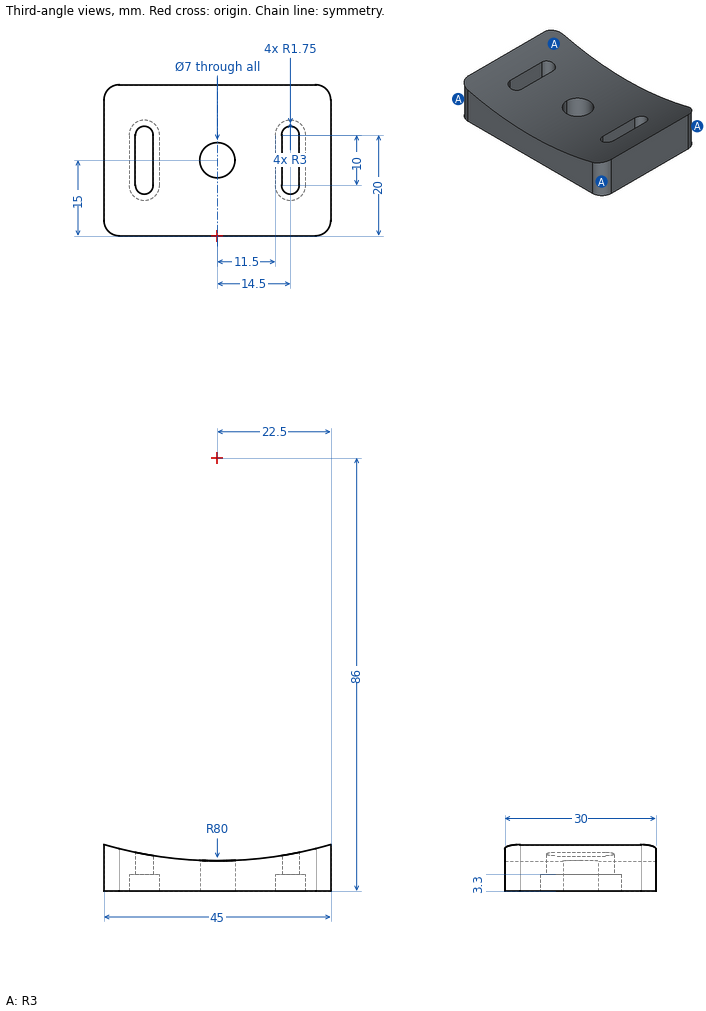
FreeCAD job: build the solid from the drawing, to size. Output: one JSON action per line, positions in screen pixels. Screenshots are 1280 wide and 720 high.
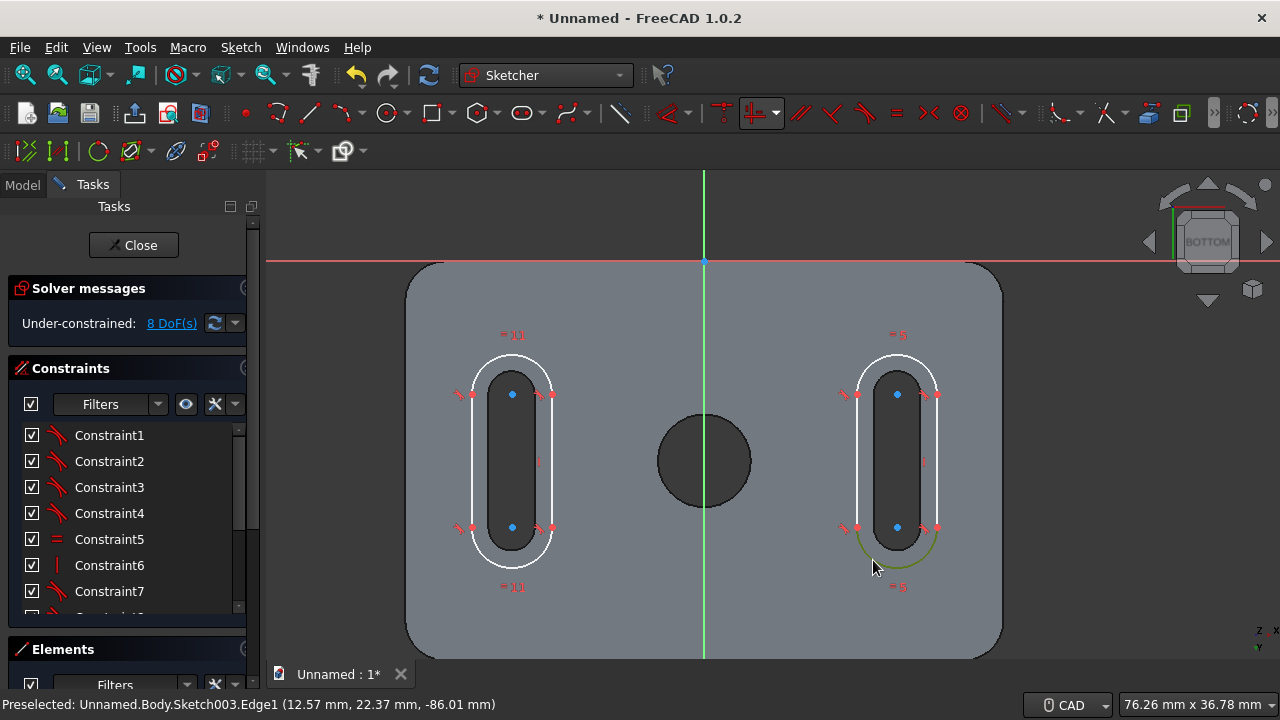
{"action": "left_click", "coordinate": [488, 560]}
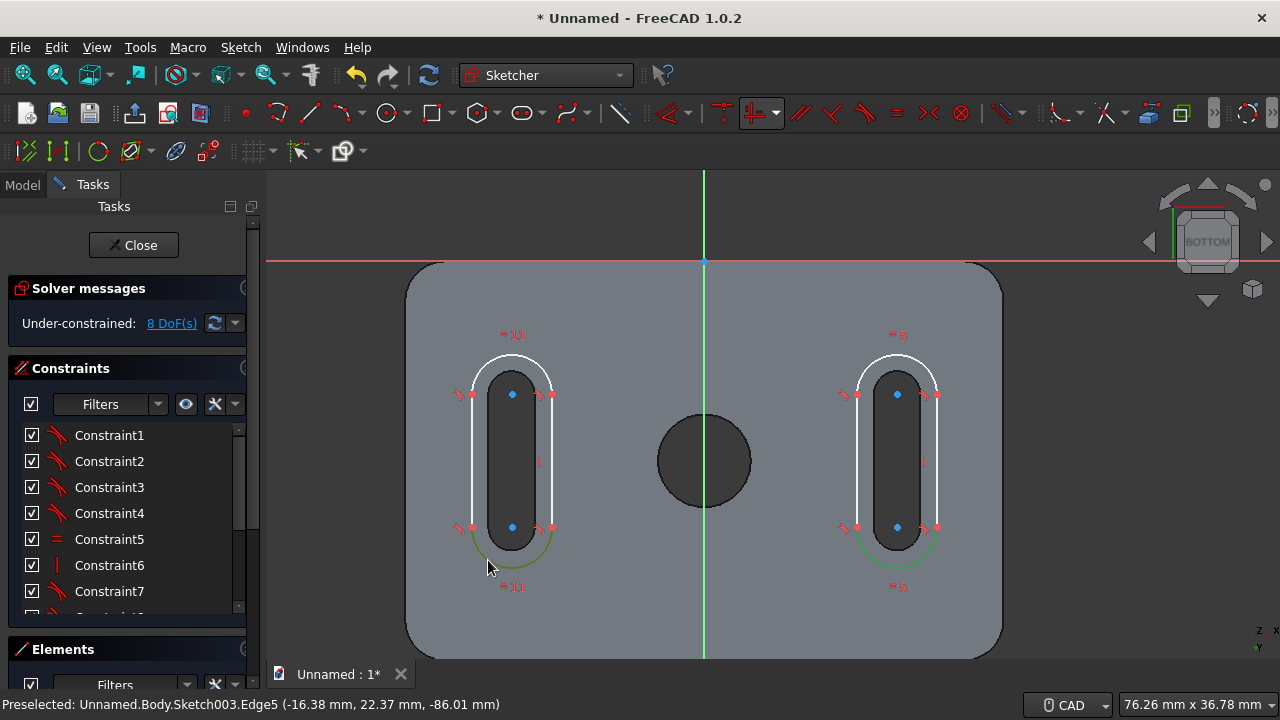
{"action": "left_click", "coordinate": [898, 114]}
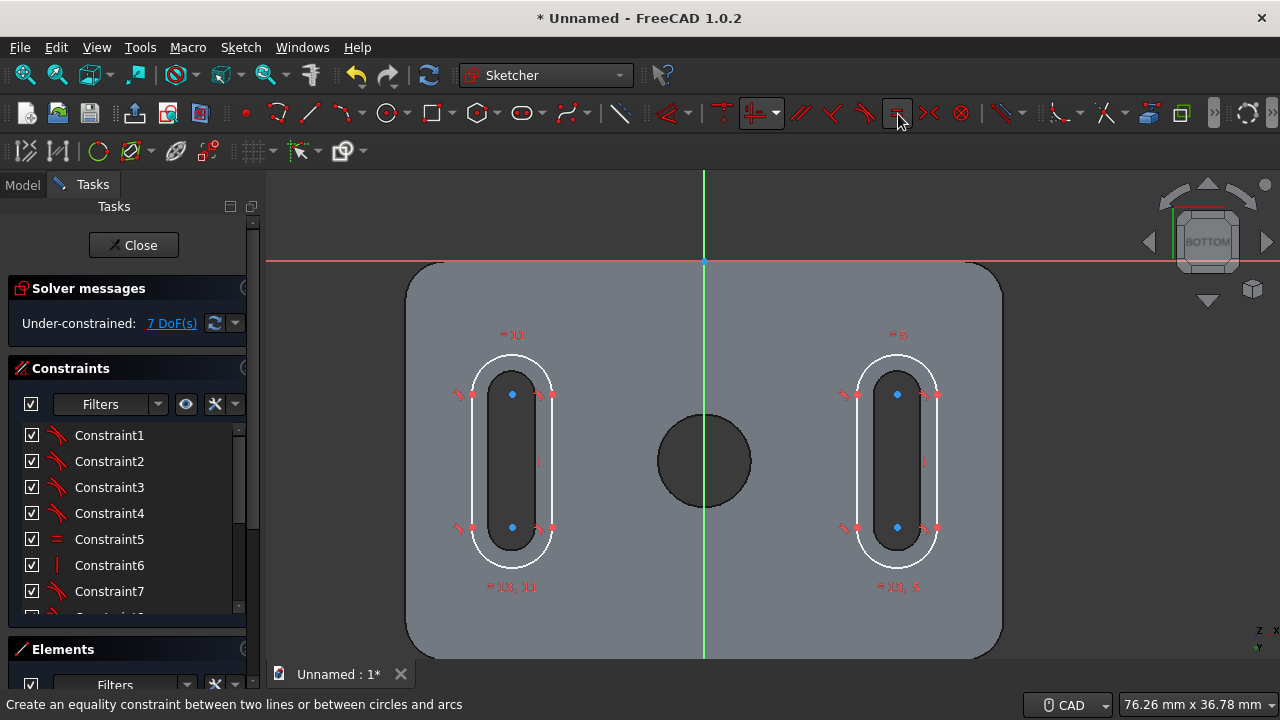
{"action": "left_click", "coordinate": [897, 528]}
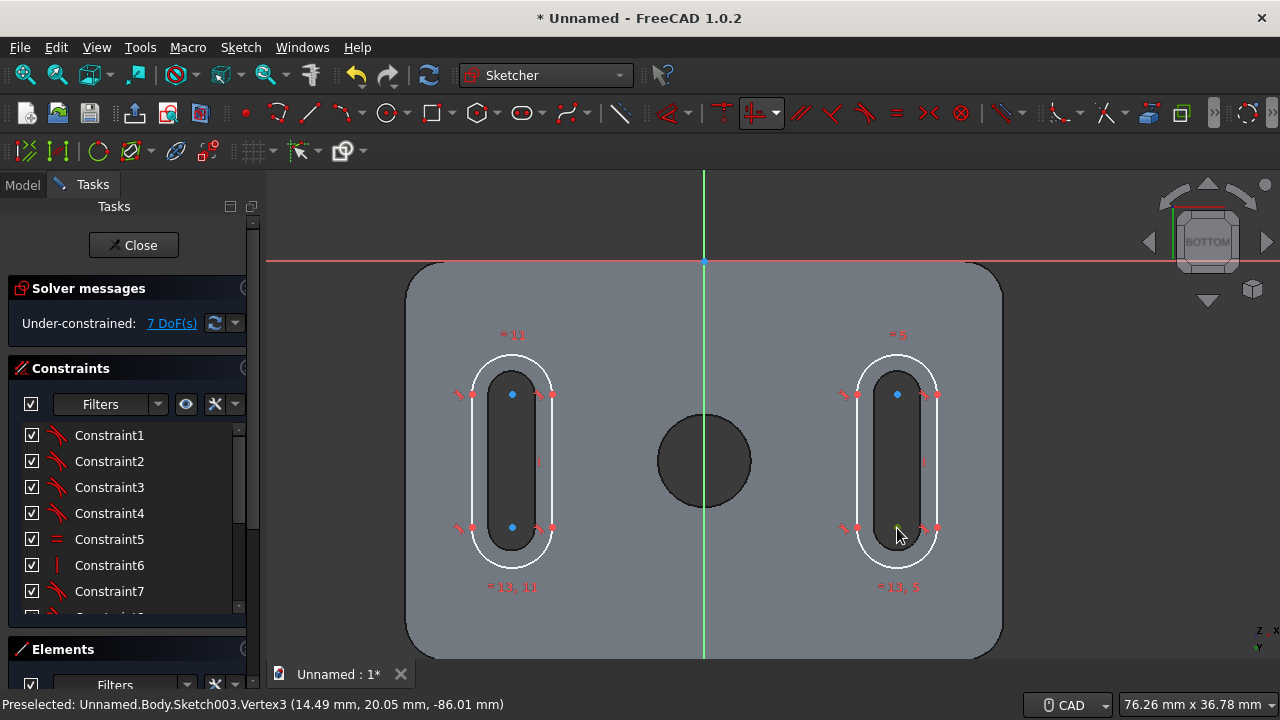
{"action": "left_click", "coordinate": [512, 528]}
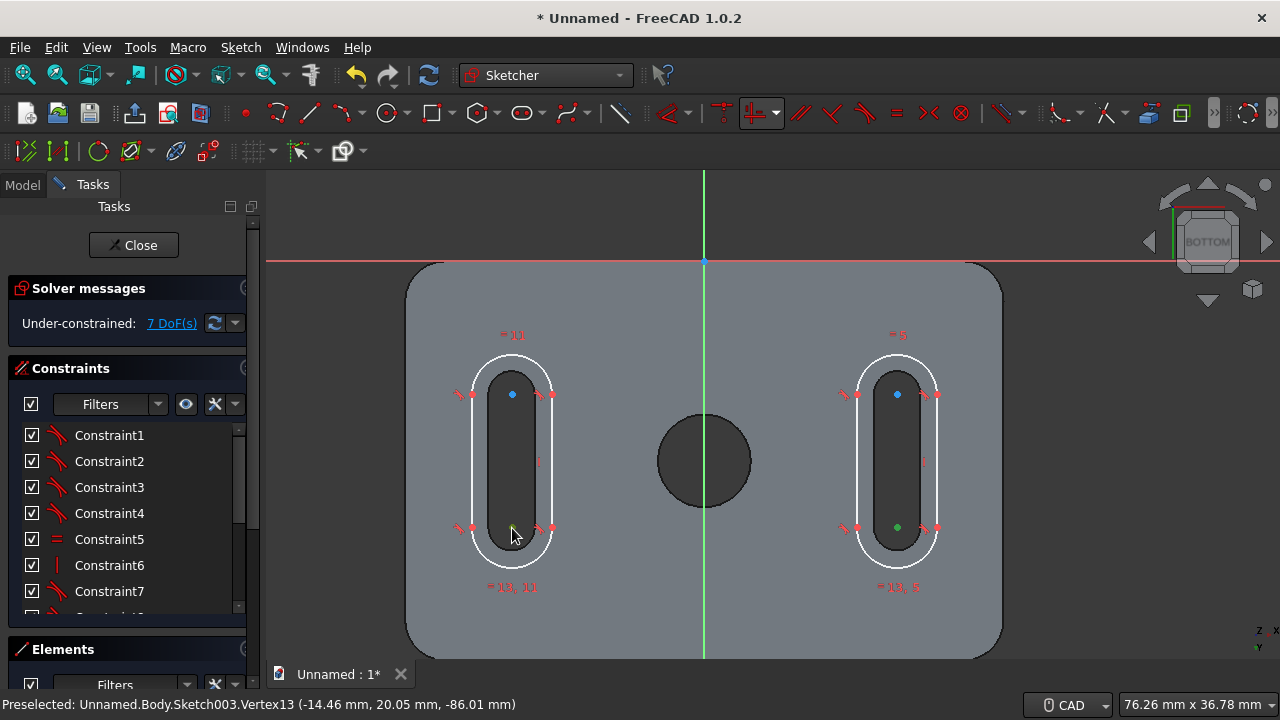
{"action": "left_click", "coordinate": [704, 600]}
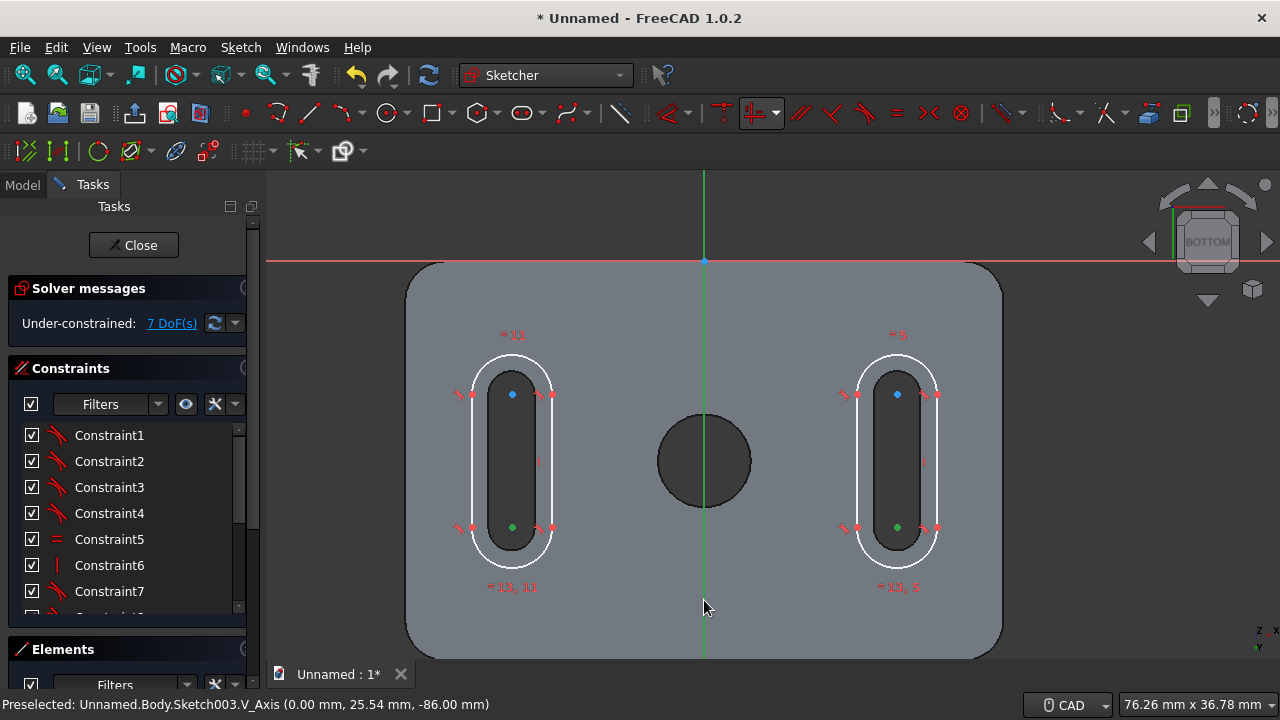
{"action": "key", "text": "s"}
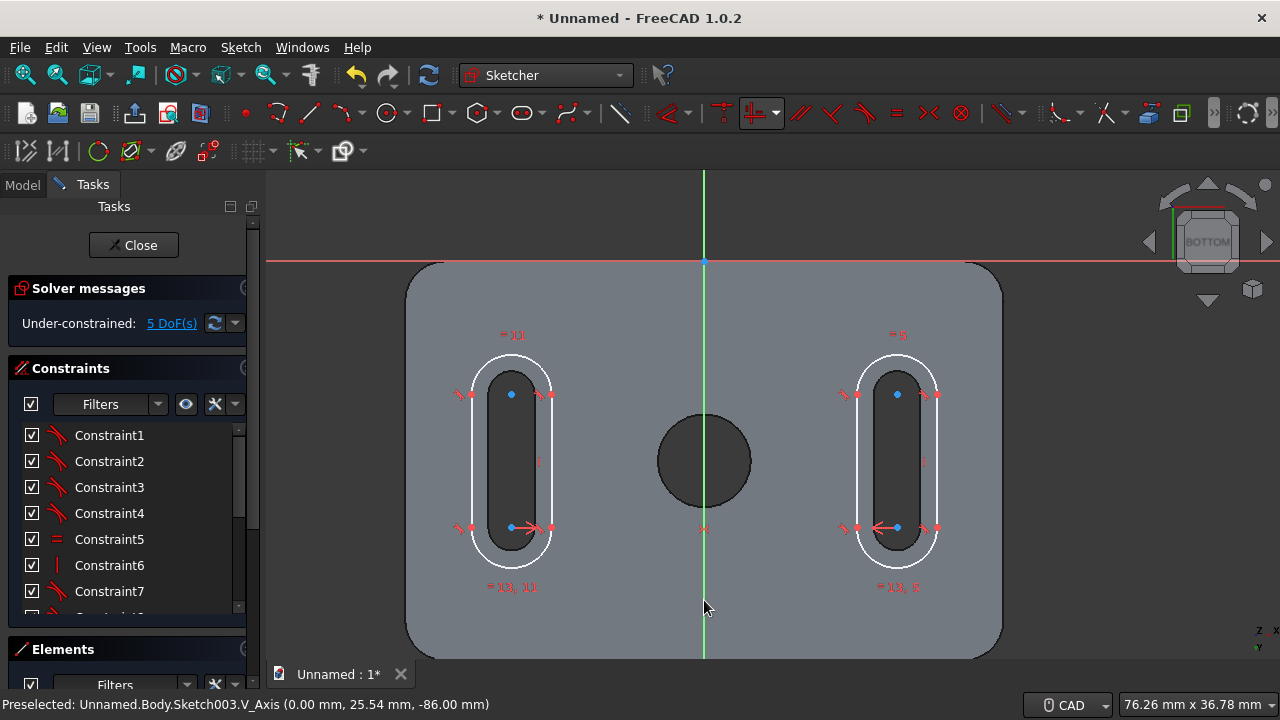
{"action": "left_click", "coordinate": [668, 114]}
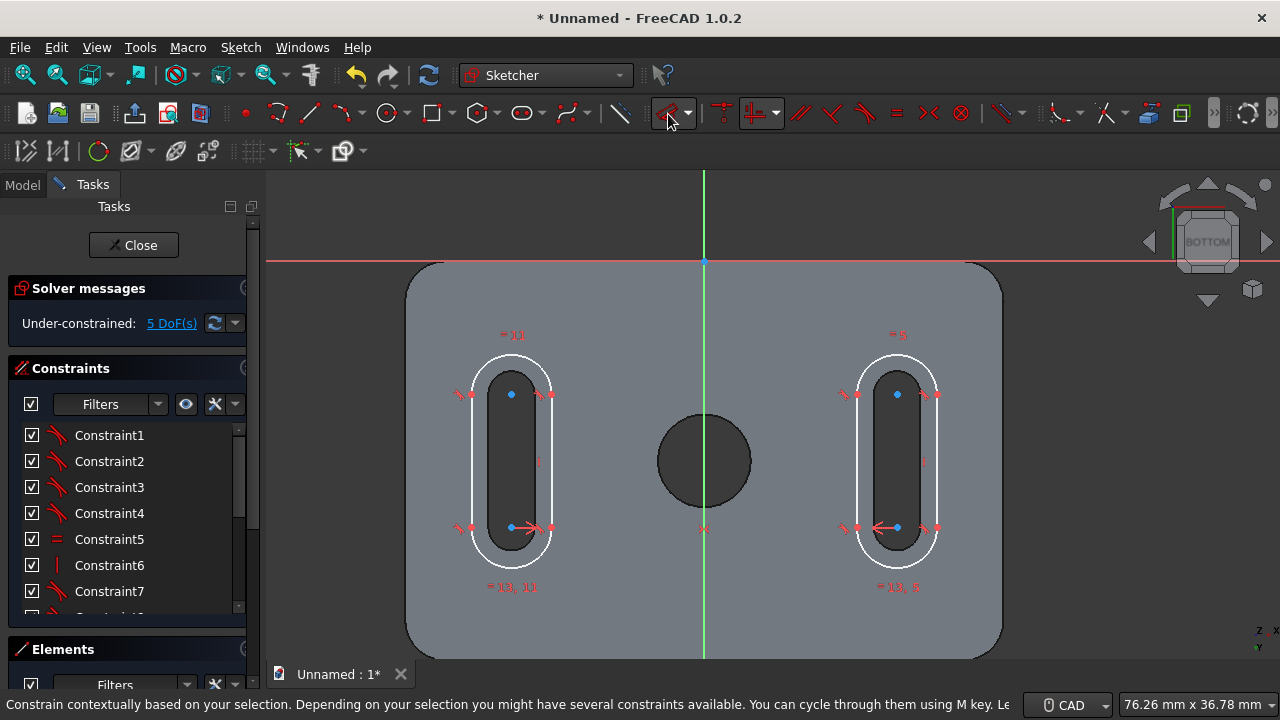
{"action": "left_click", "coordinate": [873, 560]}
{"action": "left_click", "coordinate": [854, 586]}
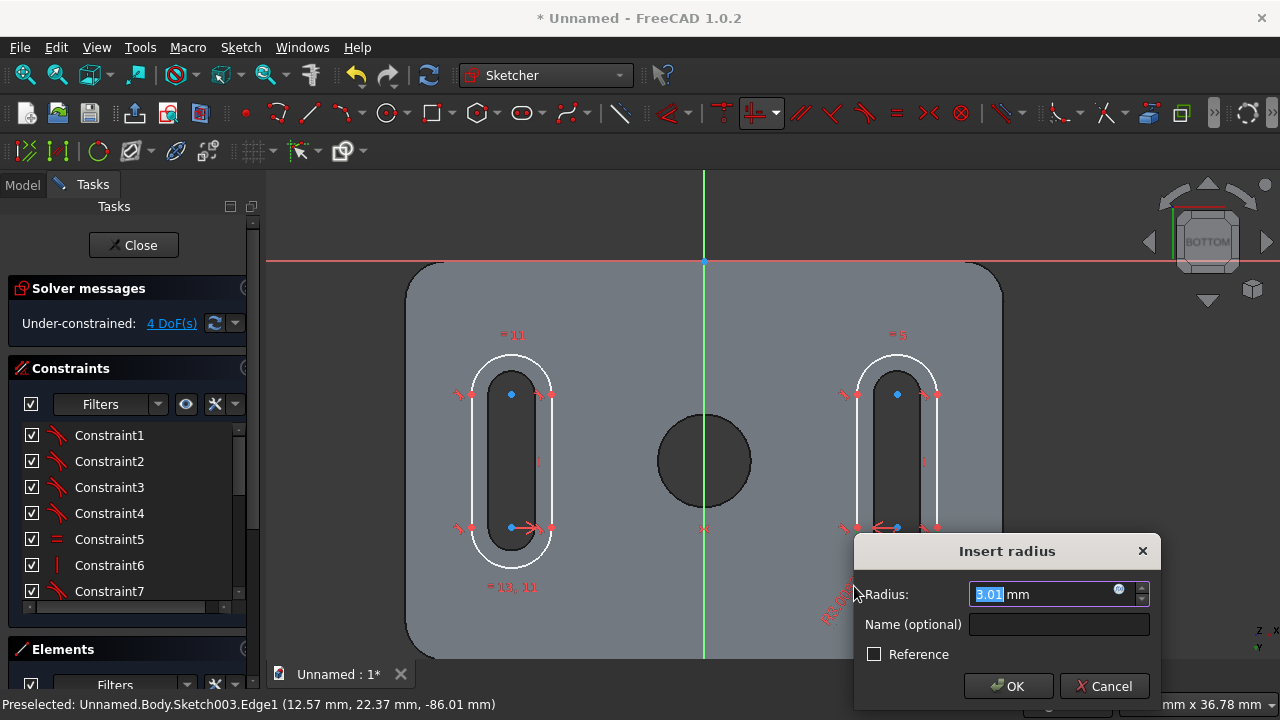
{"action": "type", "text": "3"}
{"action": "key", "text": "Return"}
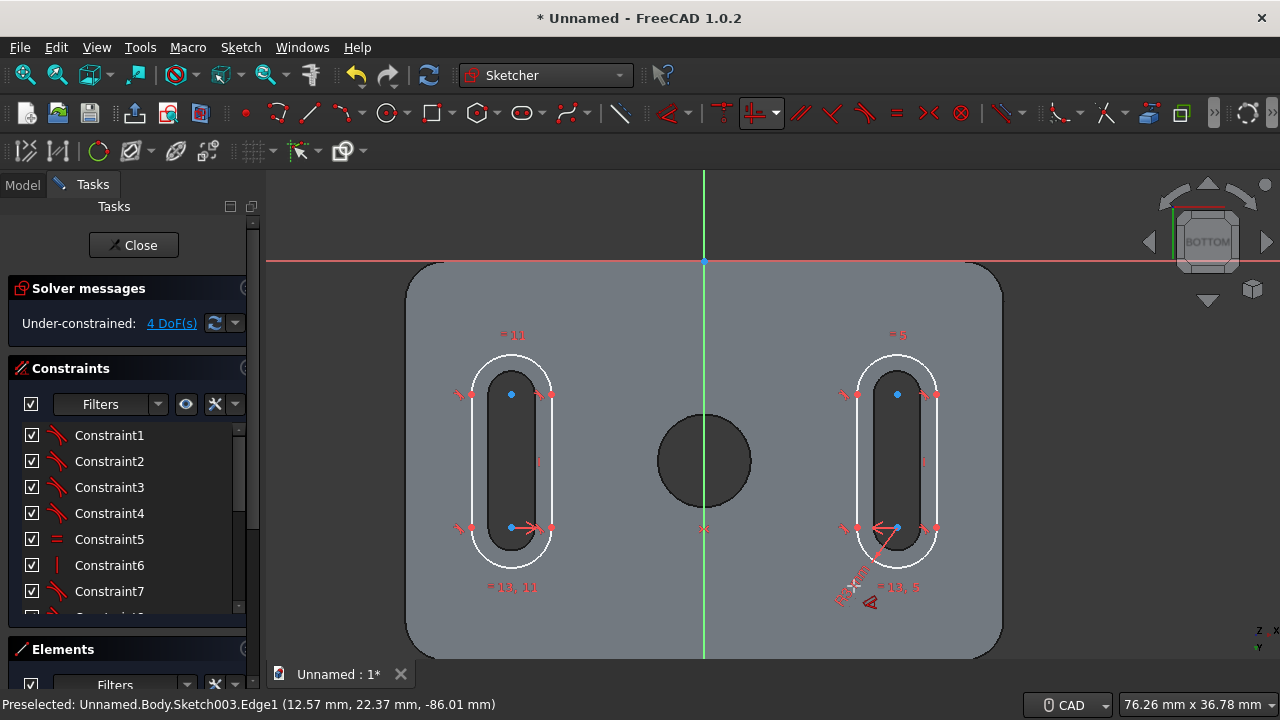
{"action": "left_click", "coordinate": [857, 488]}
{"action": "left_click", "coordinate": [891, 462]}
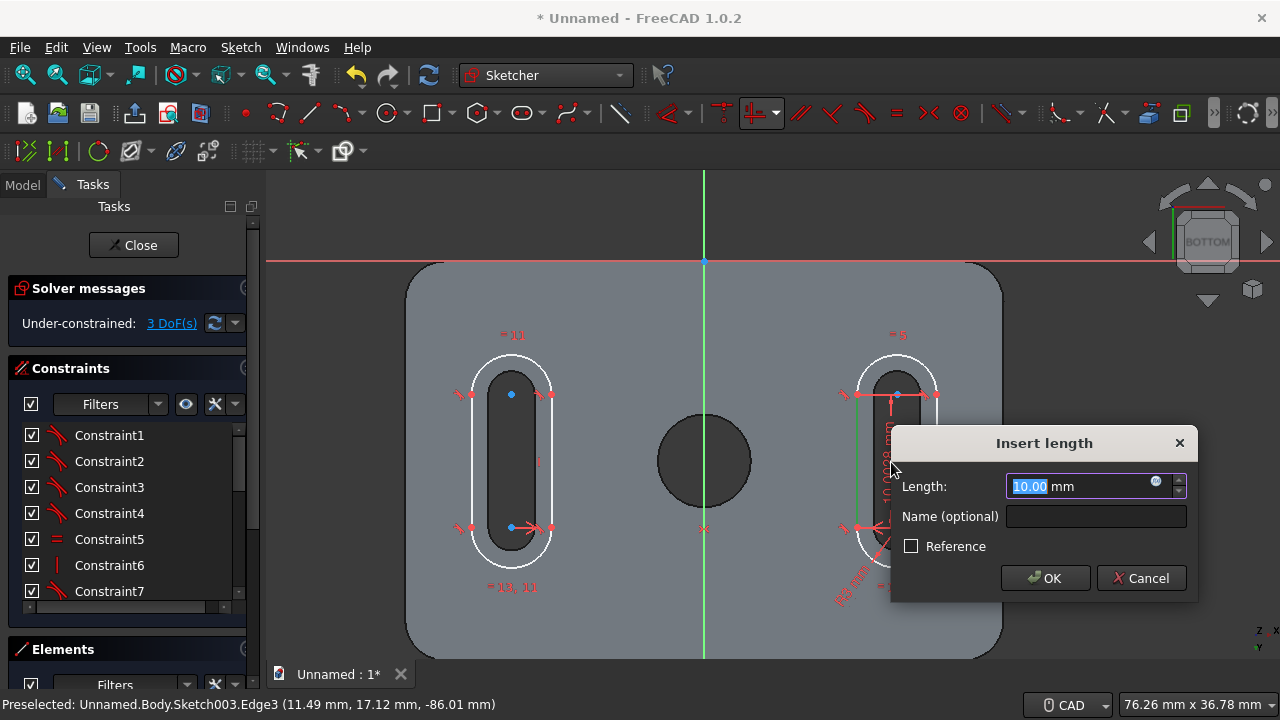
{"action": "type", "text": "10"}
{"action": "key", "text": "Return"}